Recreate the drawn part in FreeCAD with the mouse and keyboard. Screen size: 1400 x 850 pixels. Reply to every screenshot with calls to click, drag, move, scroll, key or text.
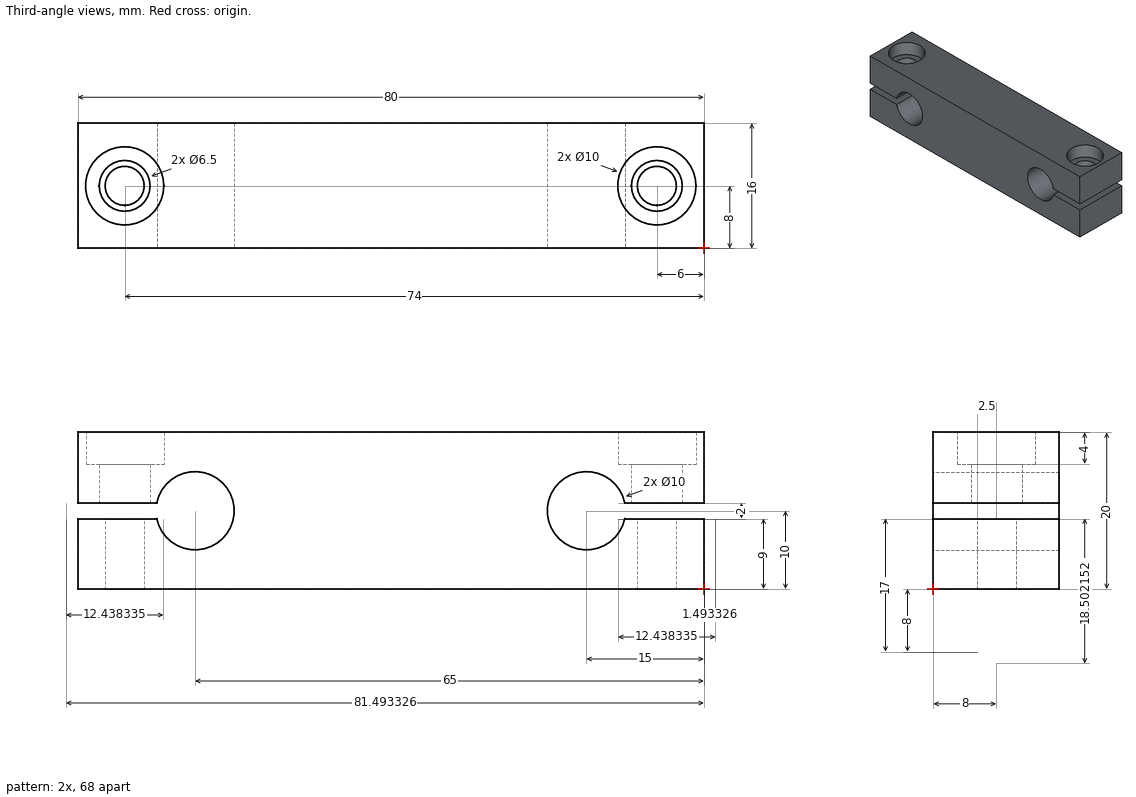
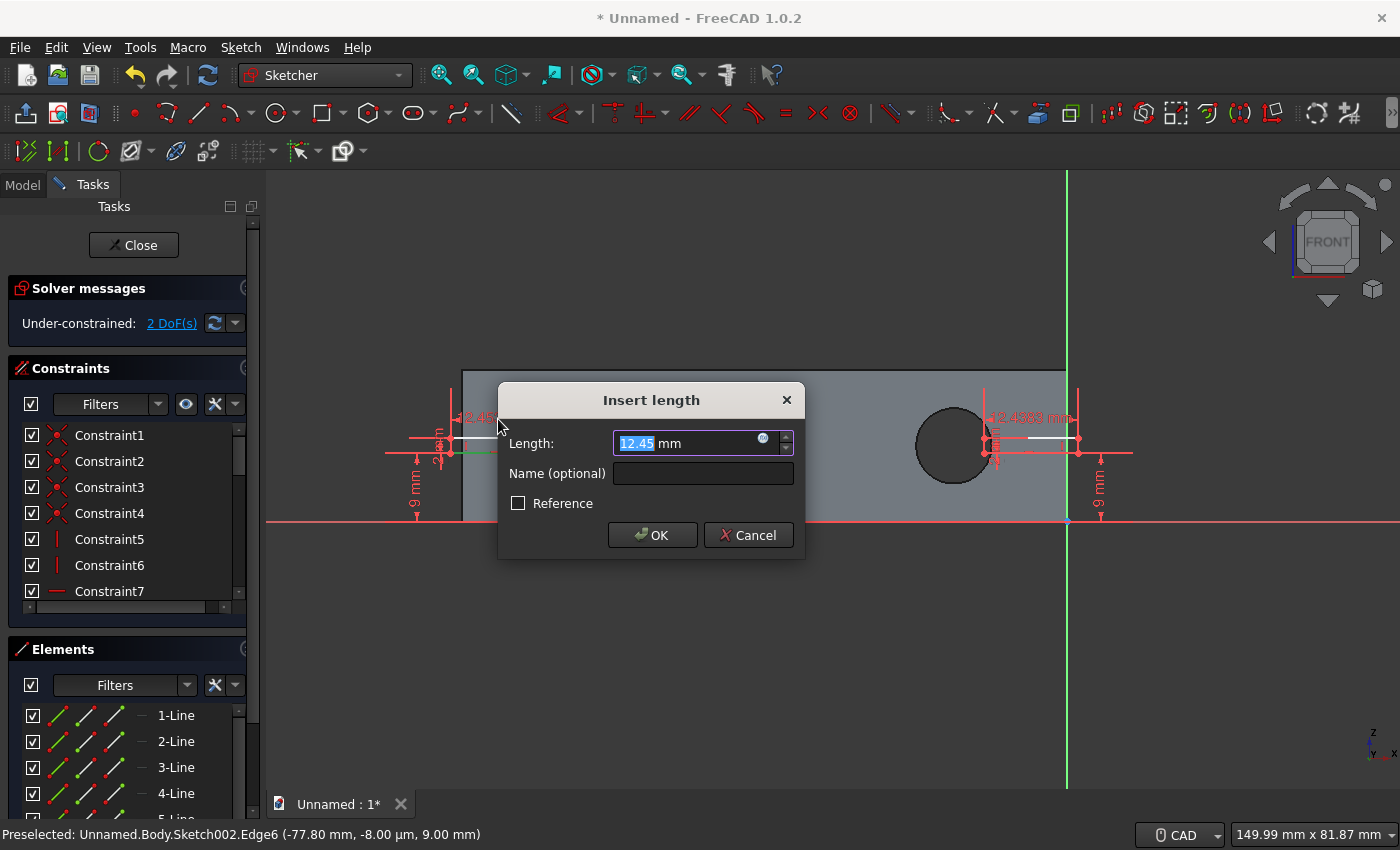
text(12.438335)
key(Return)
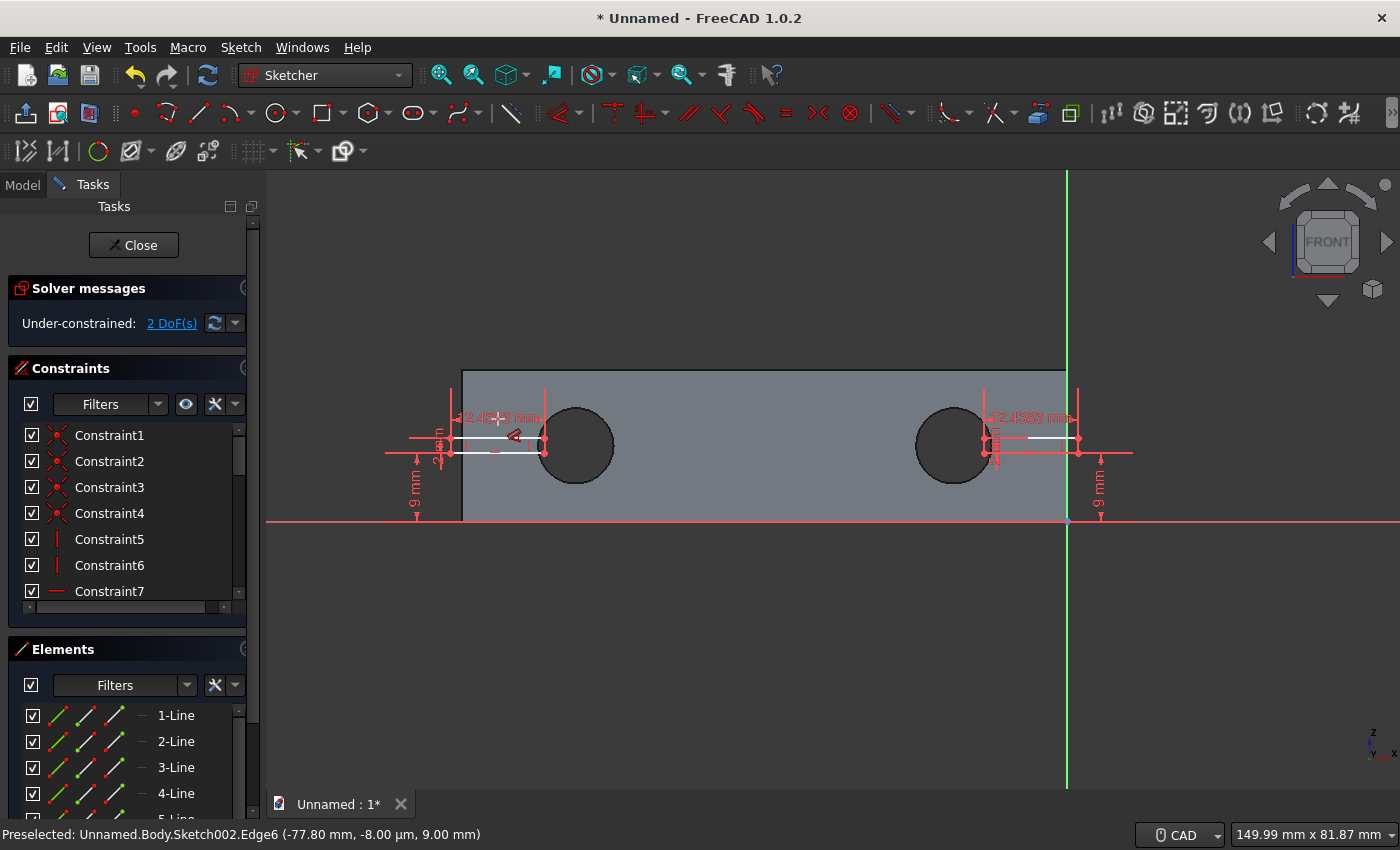
scroll(1078, 453, up, 7)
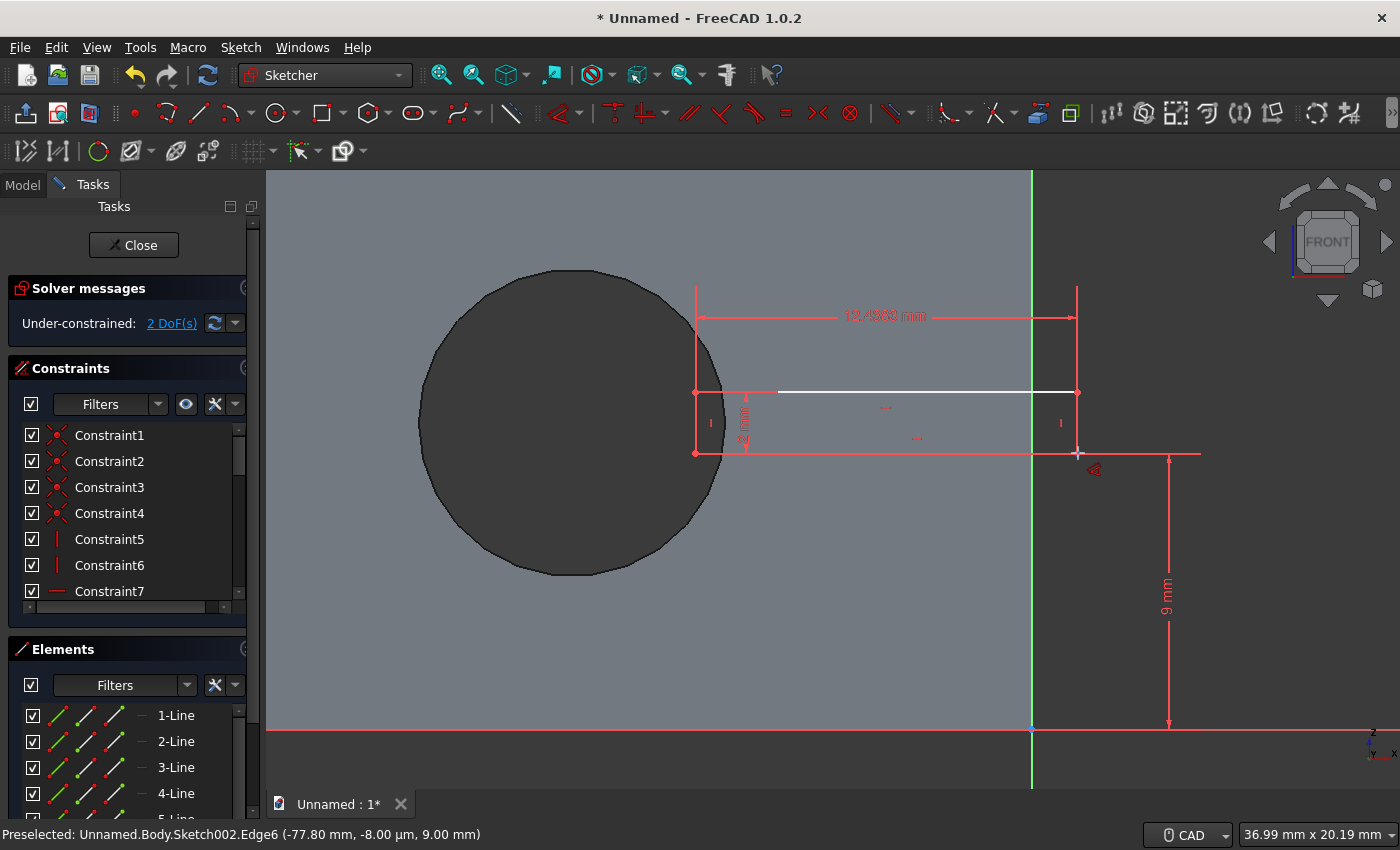
click(1077, 454)
click(1055, 420)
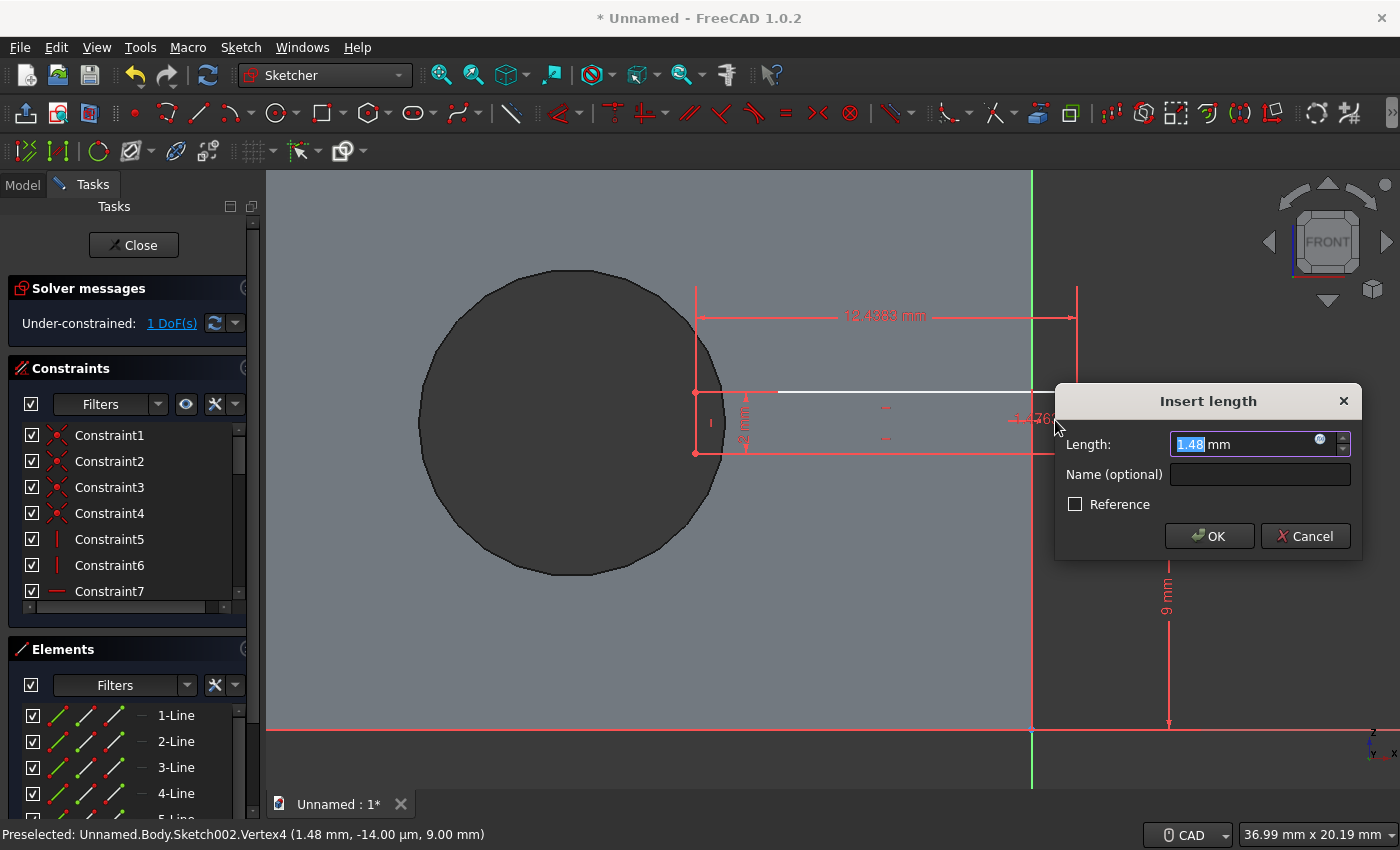
text(1.493326)
key(Return)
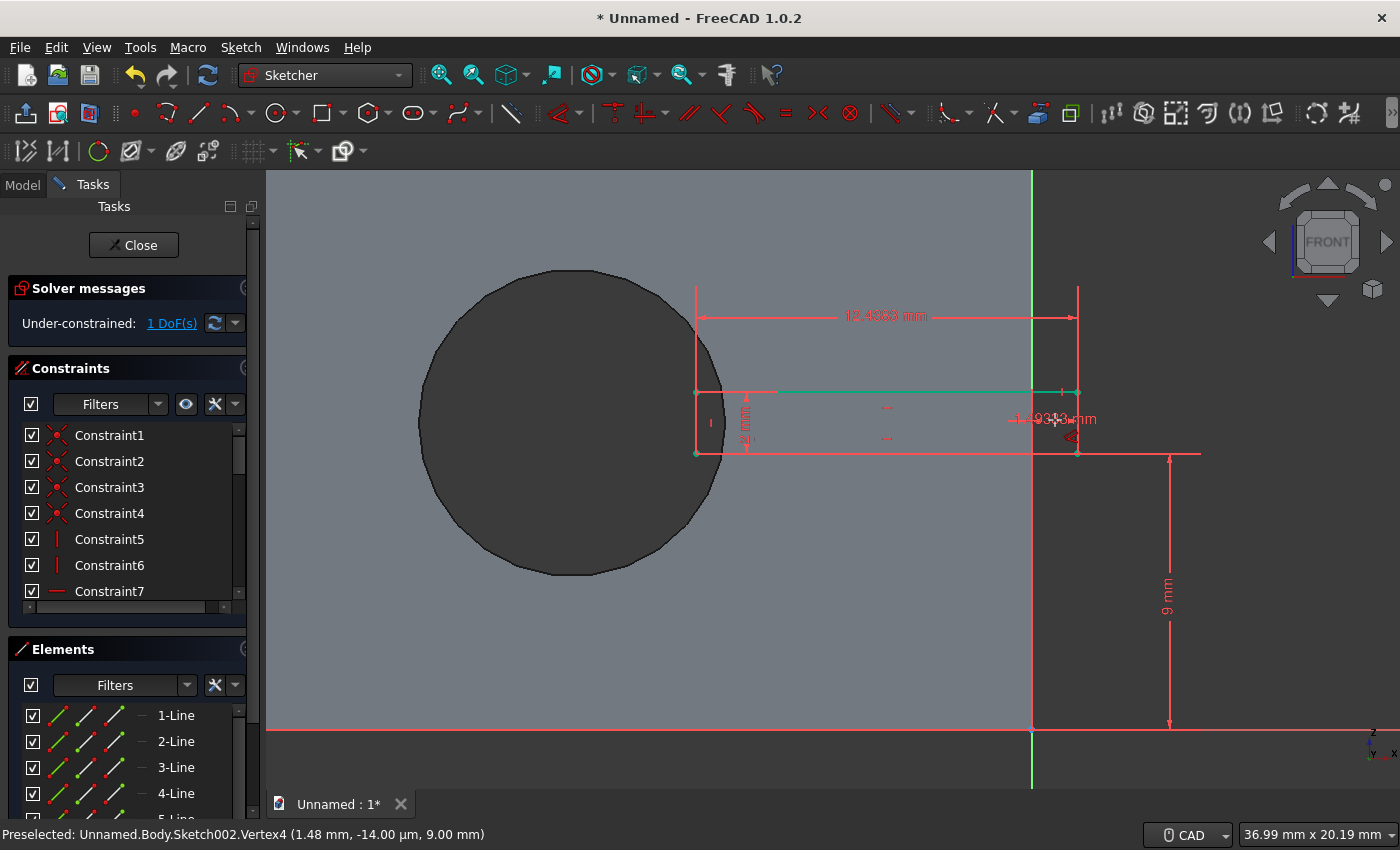
scroll(1078, 453, down, 7)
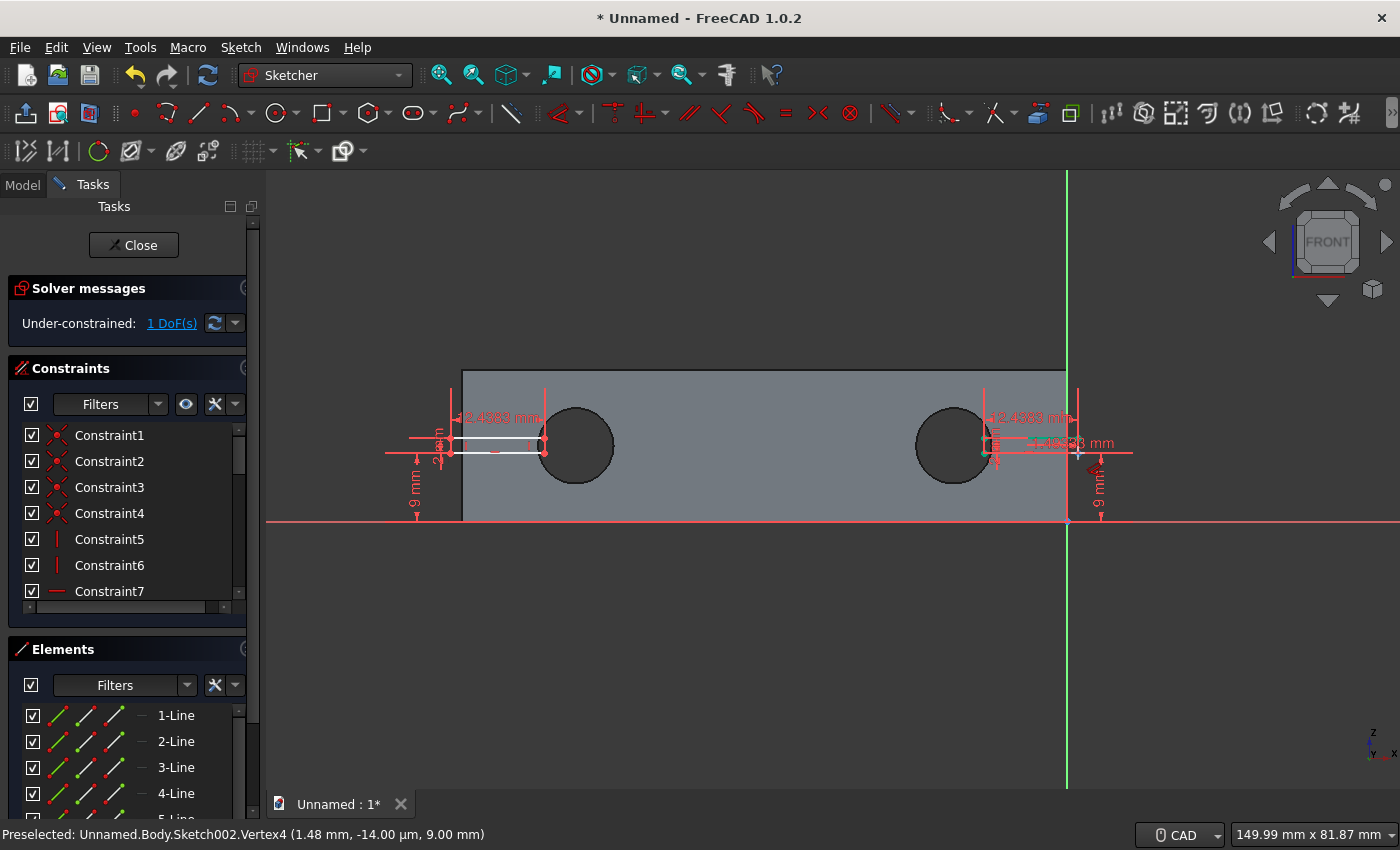
click(451, 438)
click(759, 556)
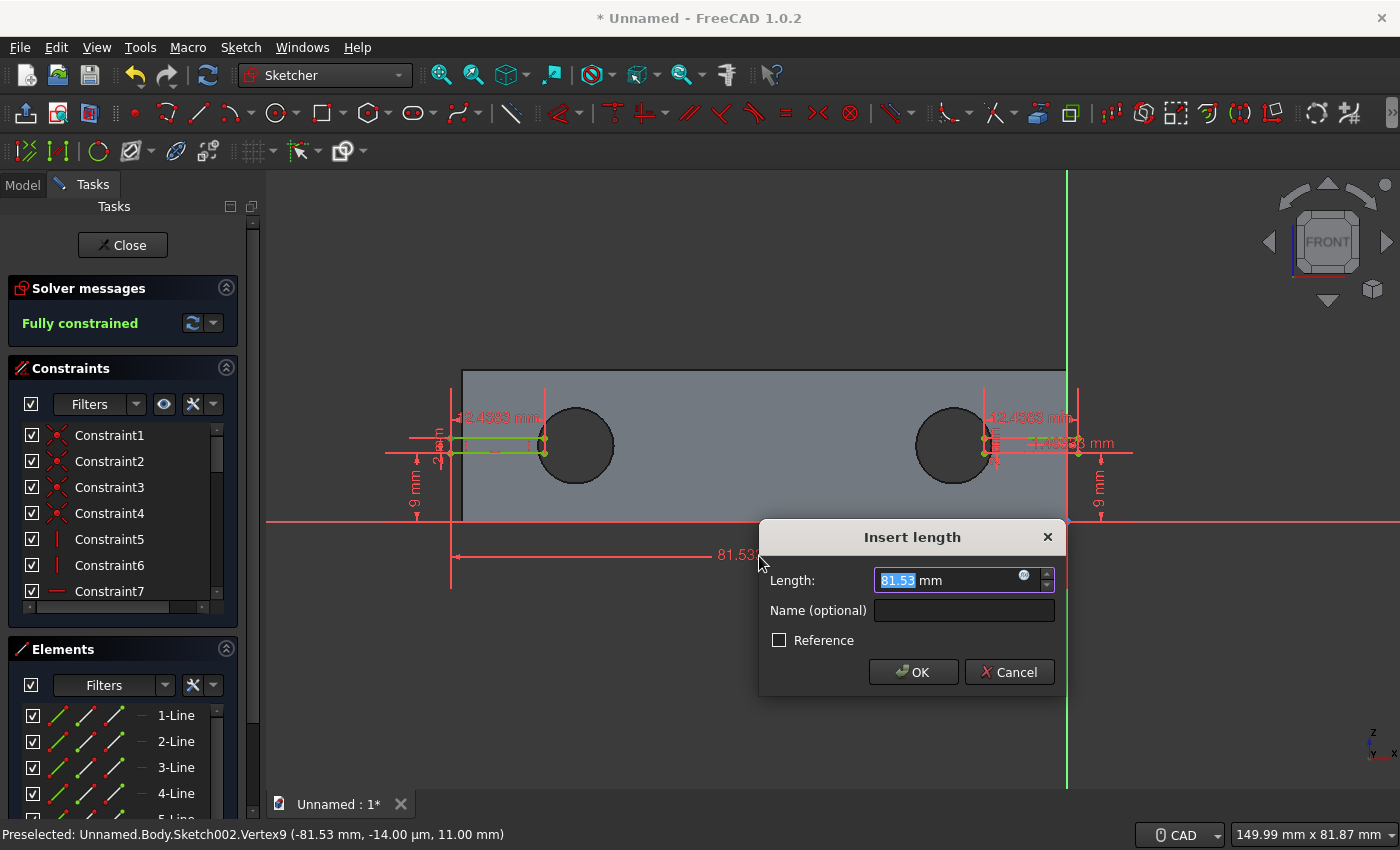
text(81.493326)
key(Return)
key(Escape)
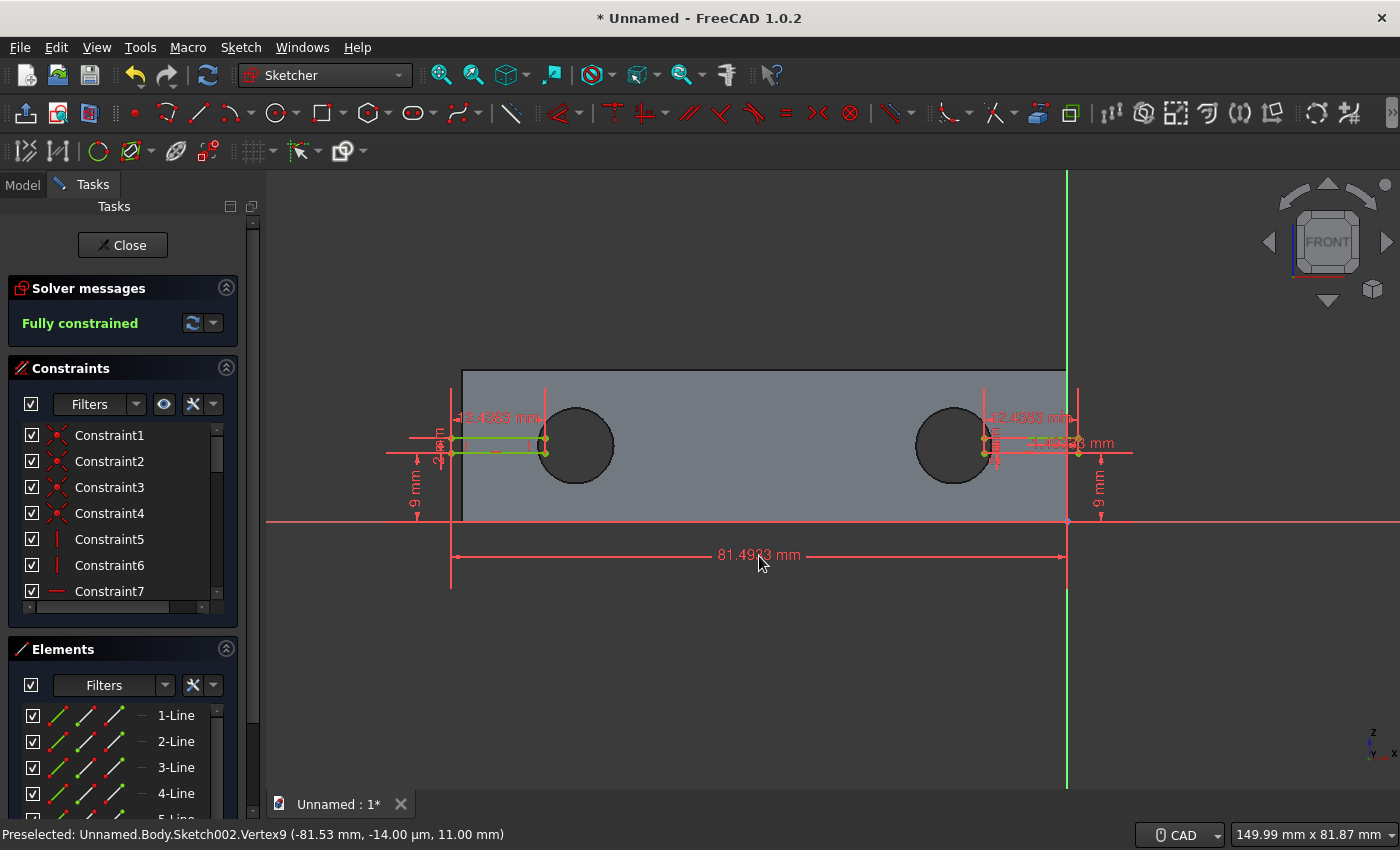
click(123, 245)